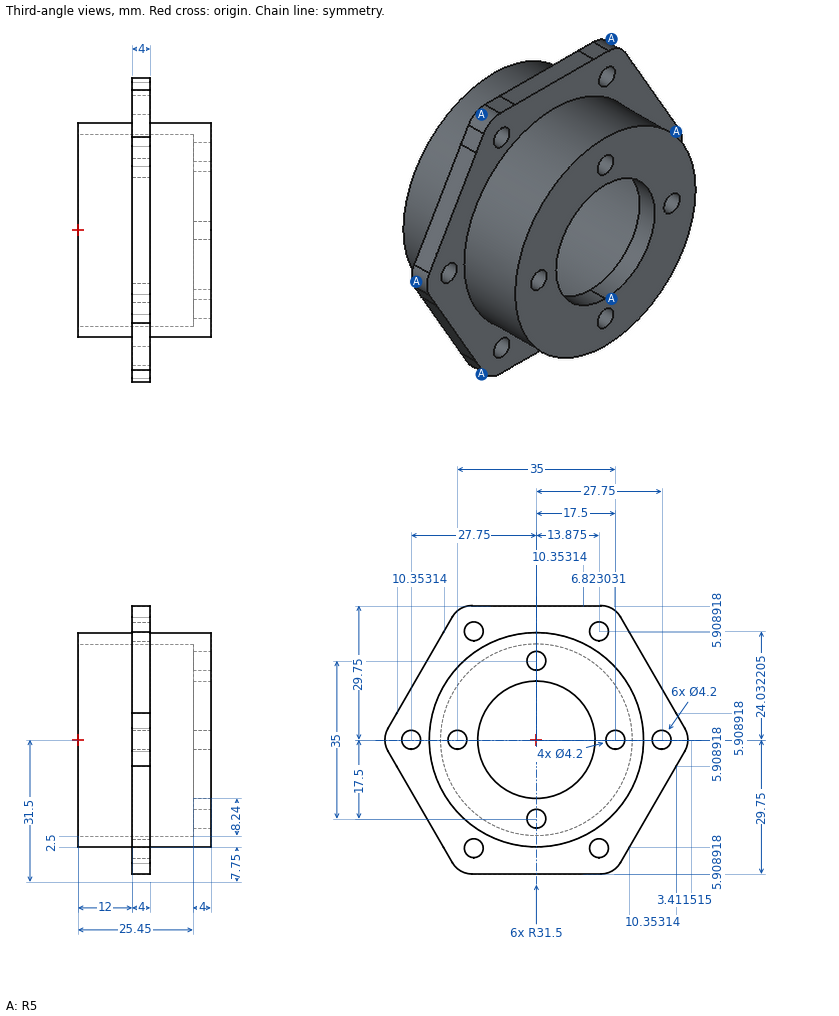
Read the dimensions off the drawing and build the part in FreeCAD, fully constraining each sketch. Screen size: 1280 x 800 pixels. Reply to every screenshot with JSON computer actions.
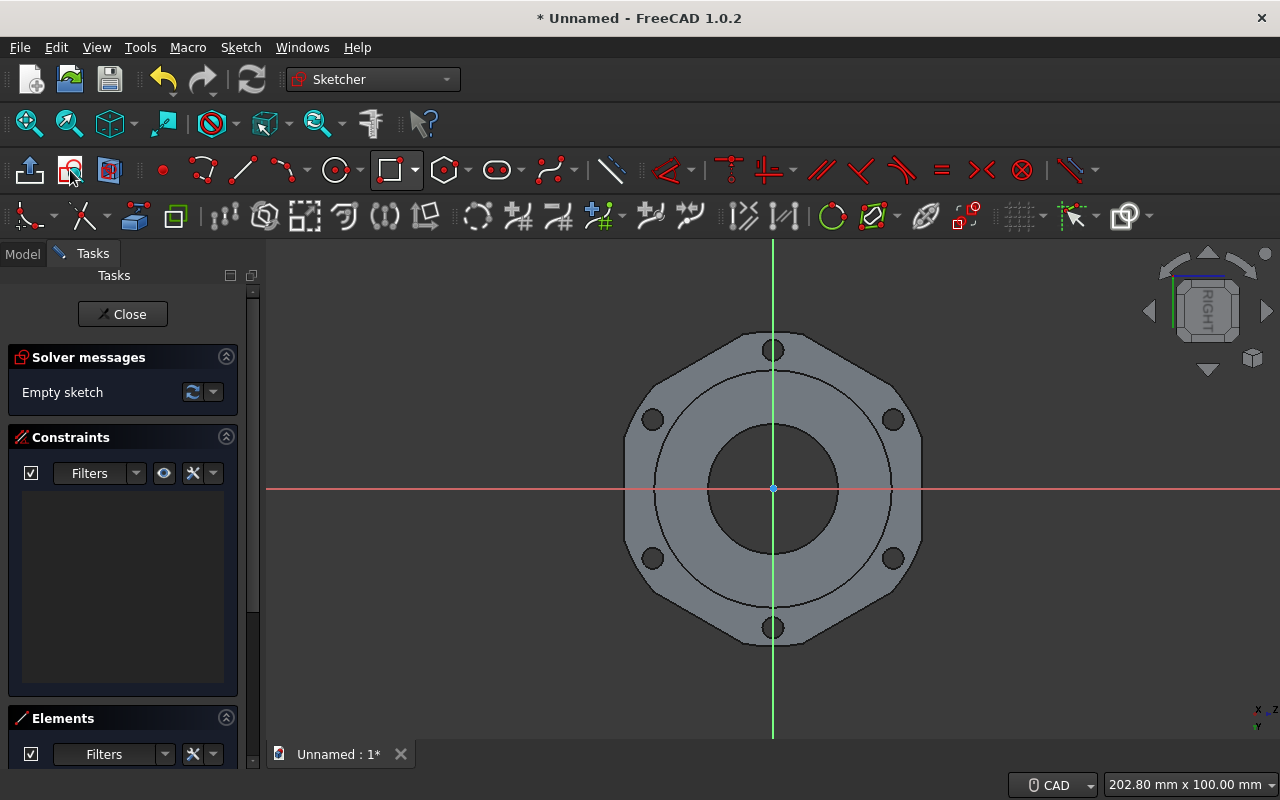
{"action": "scroll", "coordinate": [912, 489], "scroll_direction": "up", "scroll_amount": 2}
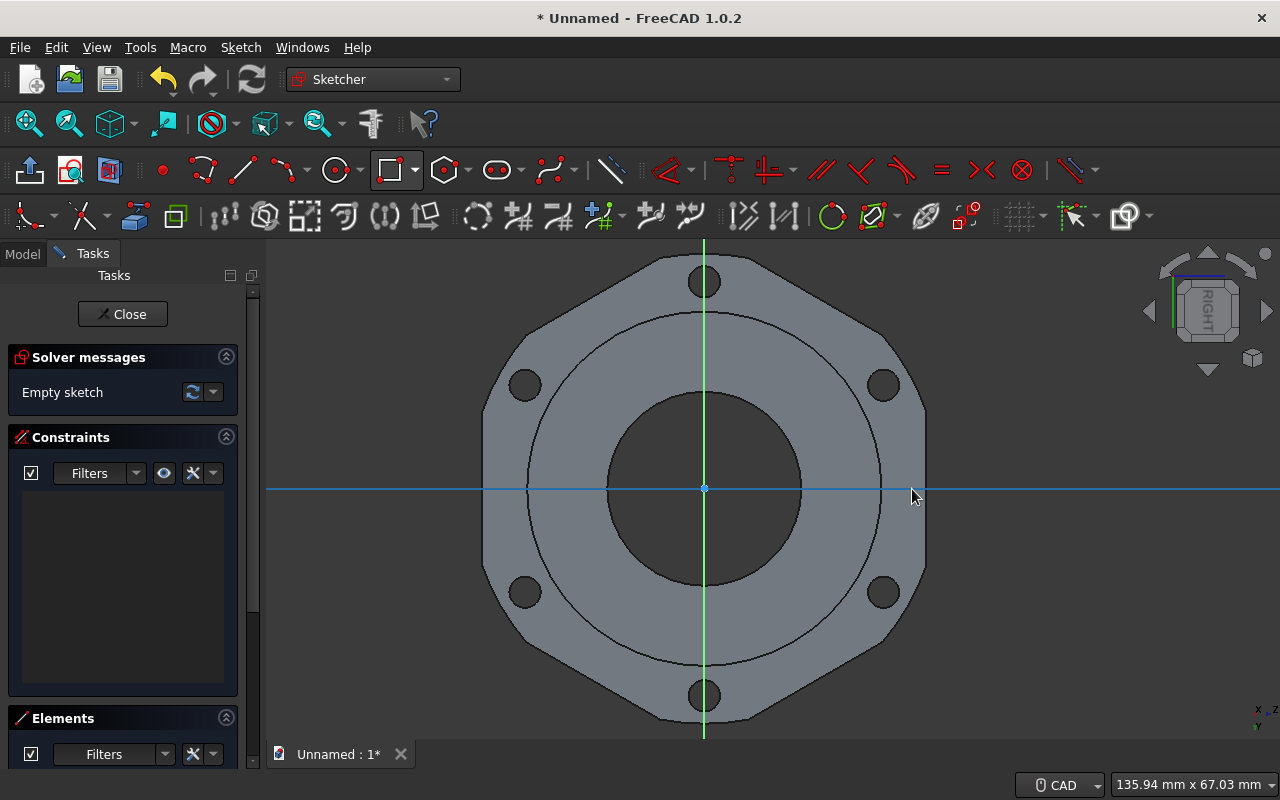
{"action": "key", "text": "g c"}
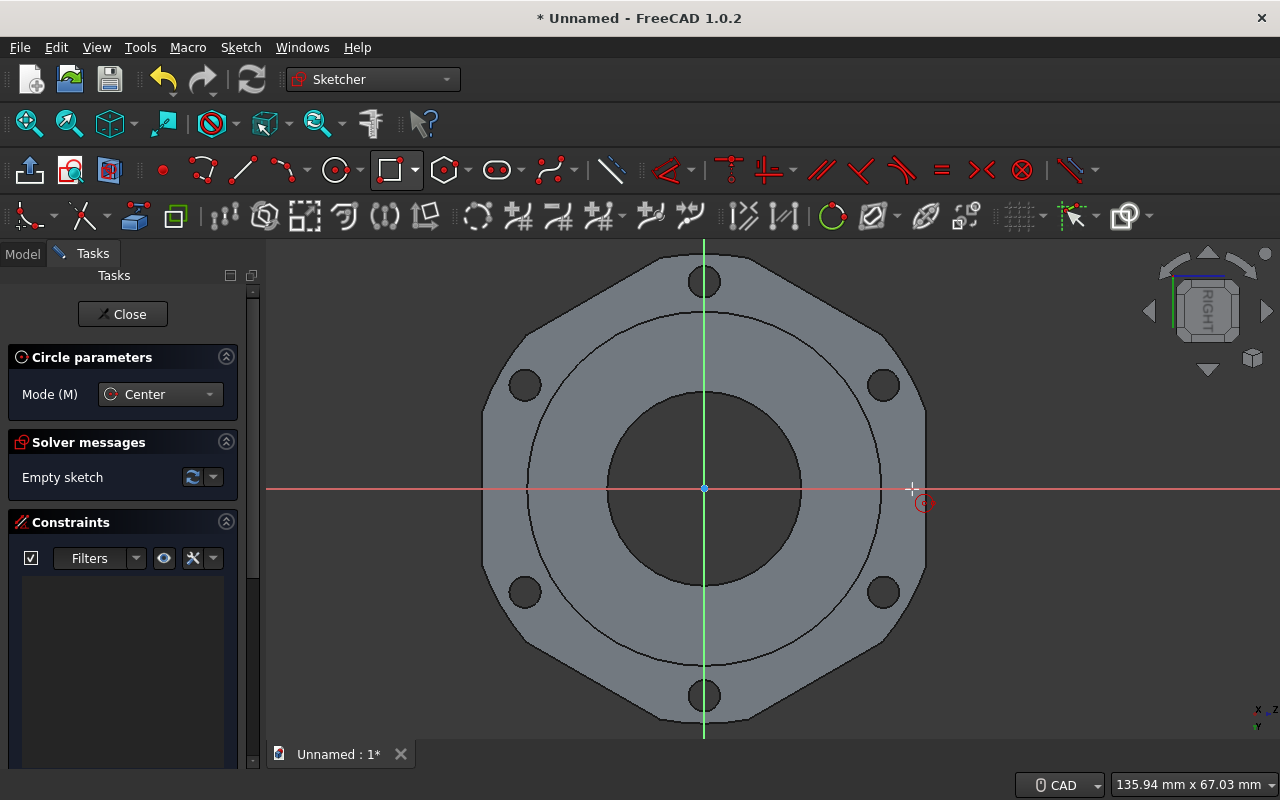
{"action": "scroll", "coordinate": [704, 619], "scroll_direction": "up", "scroll_amount": 2}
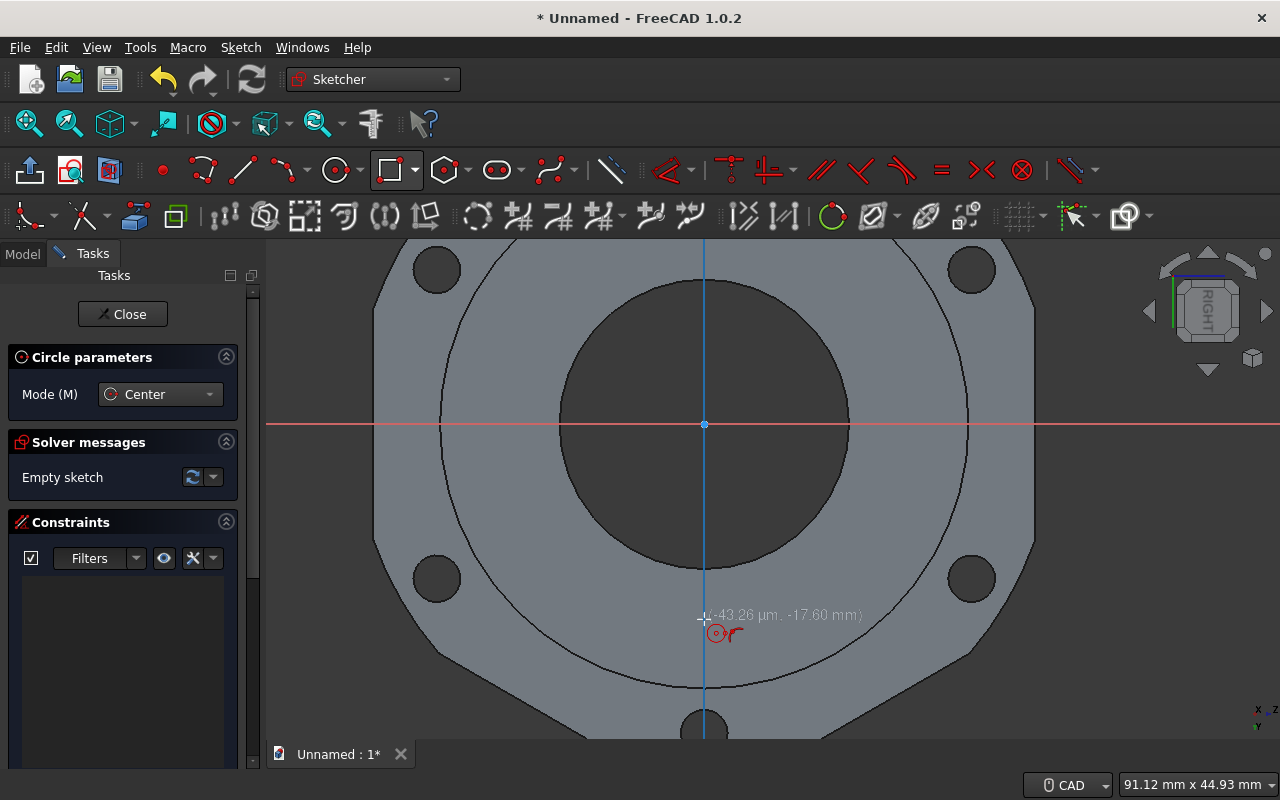
{"action": "left_click", "coordinate": [704, 619]}
{"action": "left_click", "coordinate": [721, 603]}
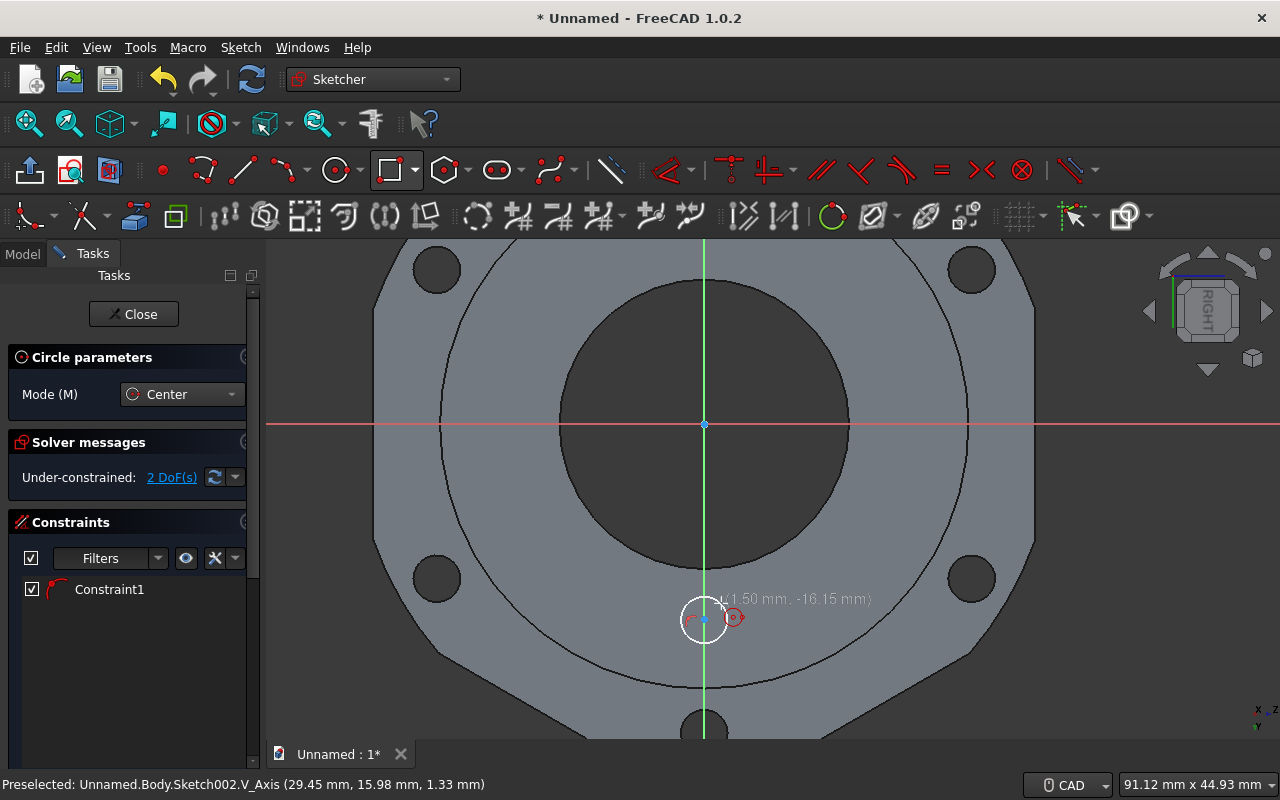
{"action": "left_click", "coordinate": [510, 424]}
{"action": "left_click", "coordinate": [526, 408]}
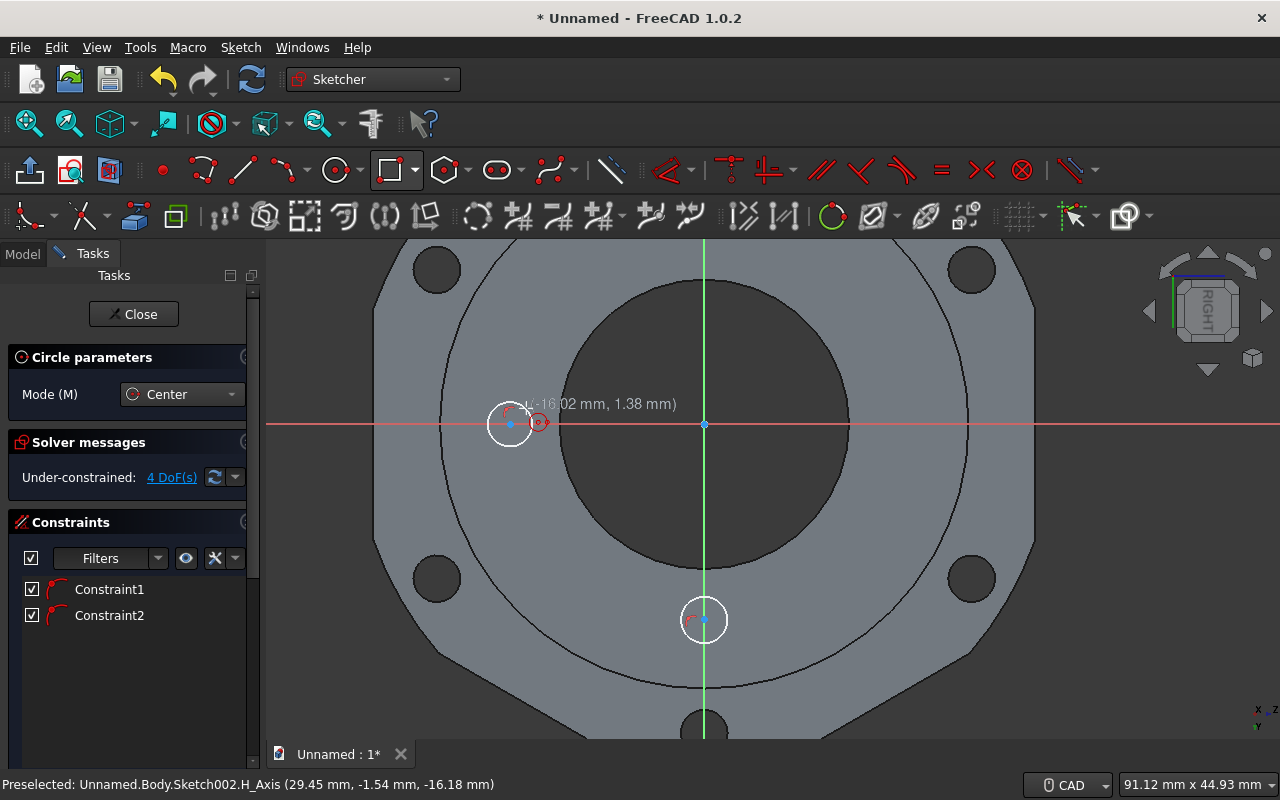
{"action": "scroll", "coordinate": [705, 621], "scroll_direction": "down", "scroll_amount": 2}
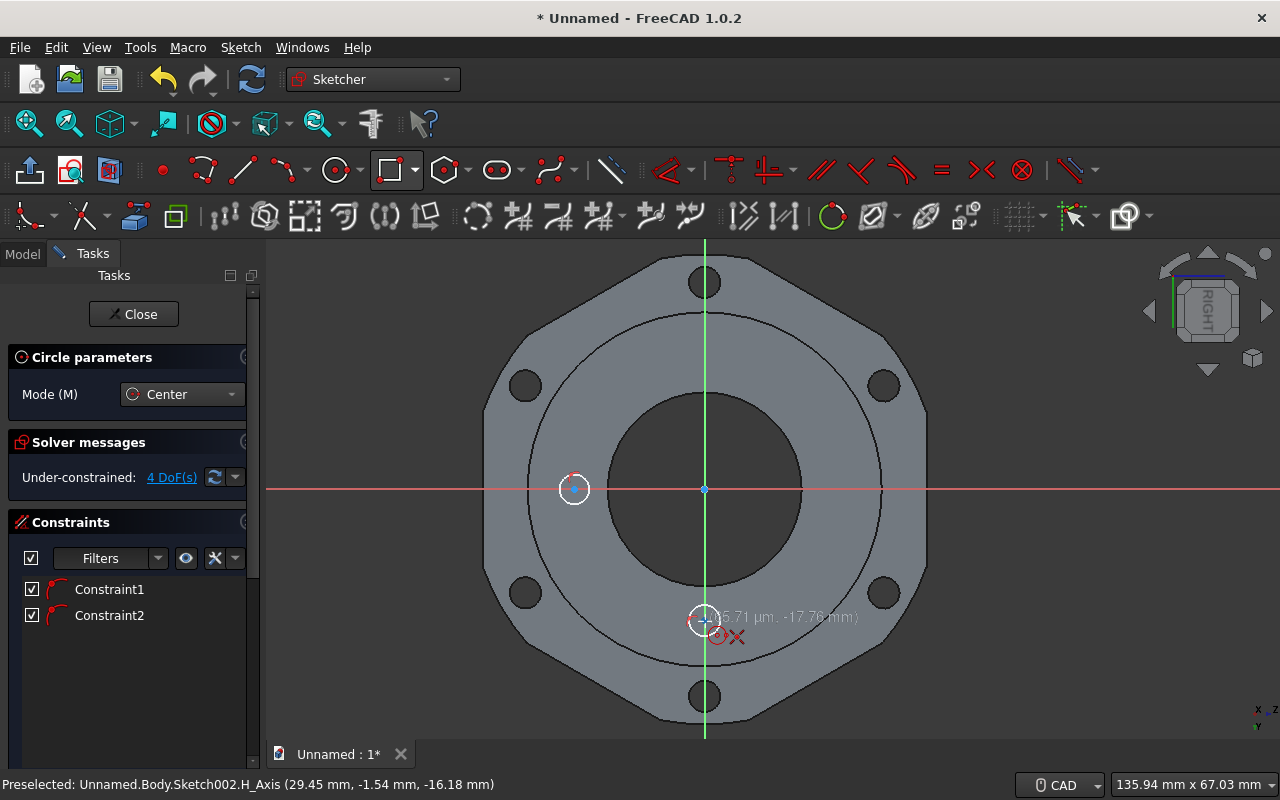
{"action": "scroll", "coordinate": [705, 359], "scroll_direction": "up", "scroll_amount": 2}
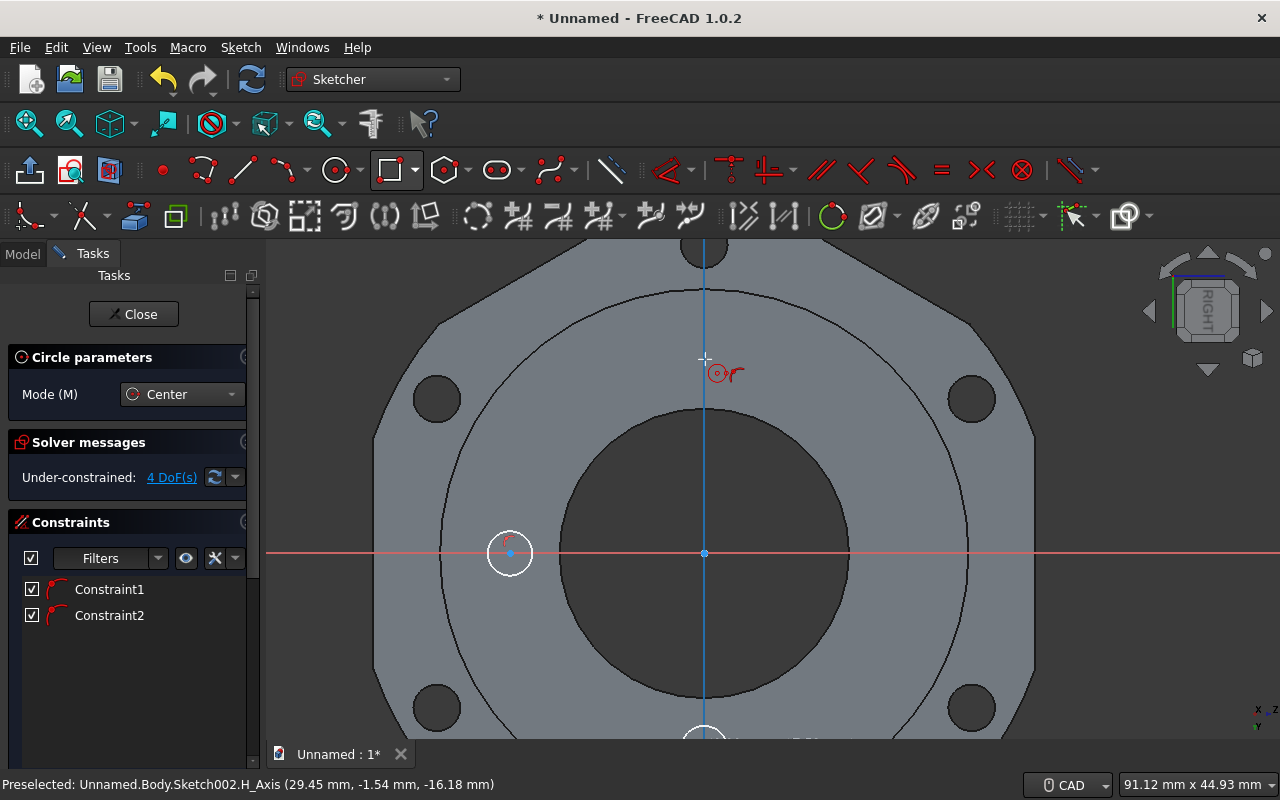
{"action": "left_click", "coordinate": [704, 359]}
{"action": "left_click", "coordinate": [721, 342]}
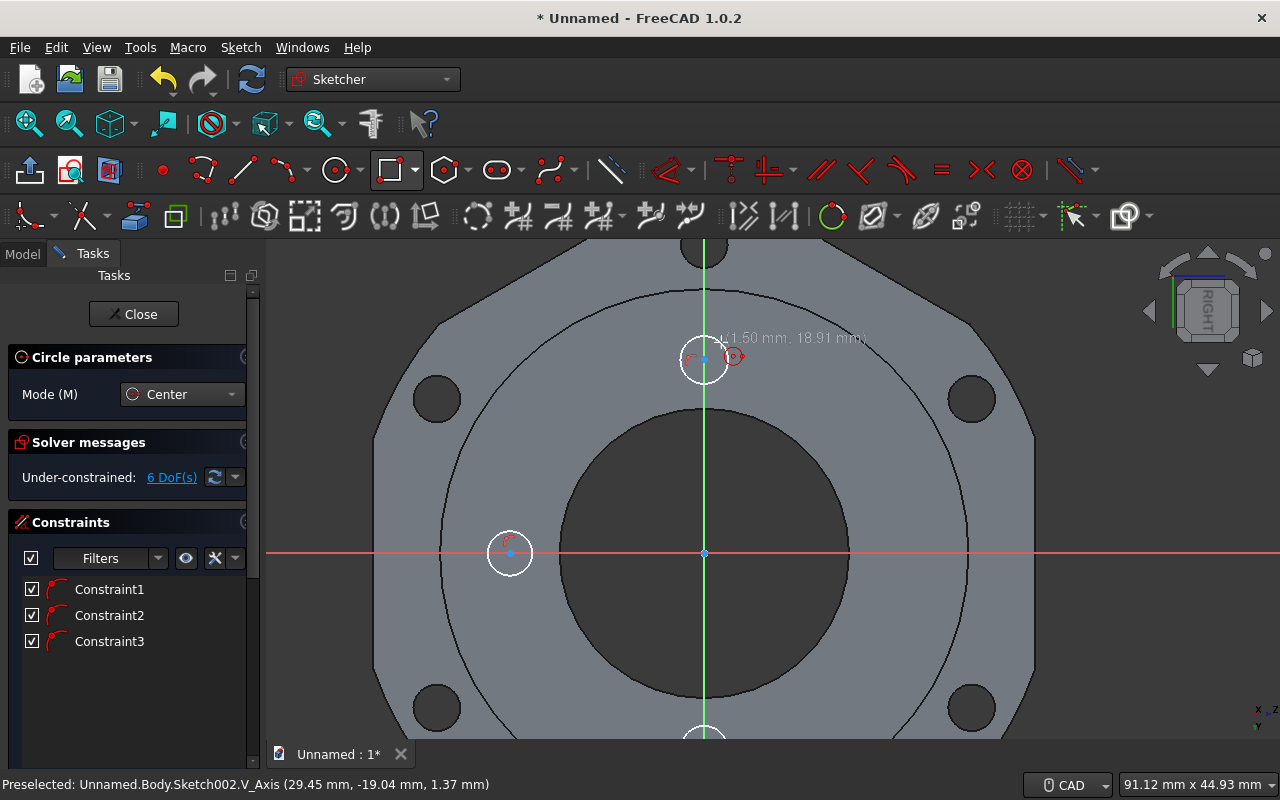
{"action": "left_click", "coordinate": [899, 553]}
{"action": "left_click", "coordinate": [916, 537]}
{"action": "key", "text": "Escape"}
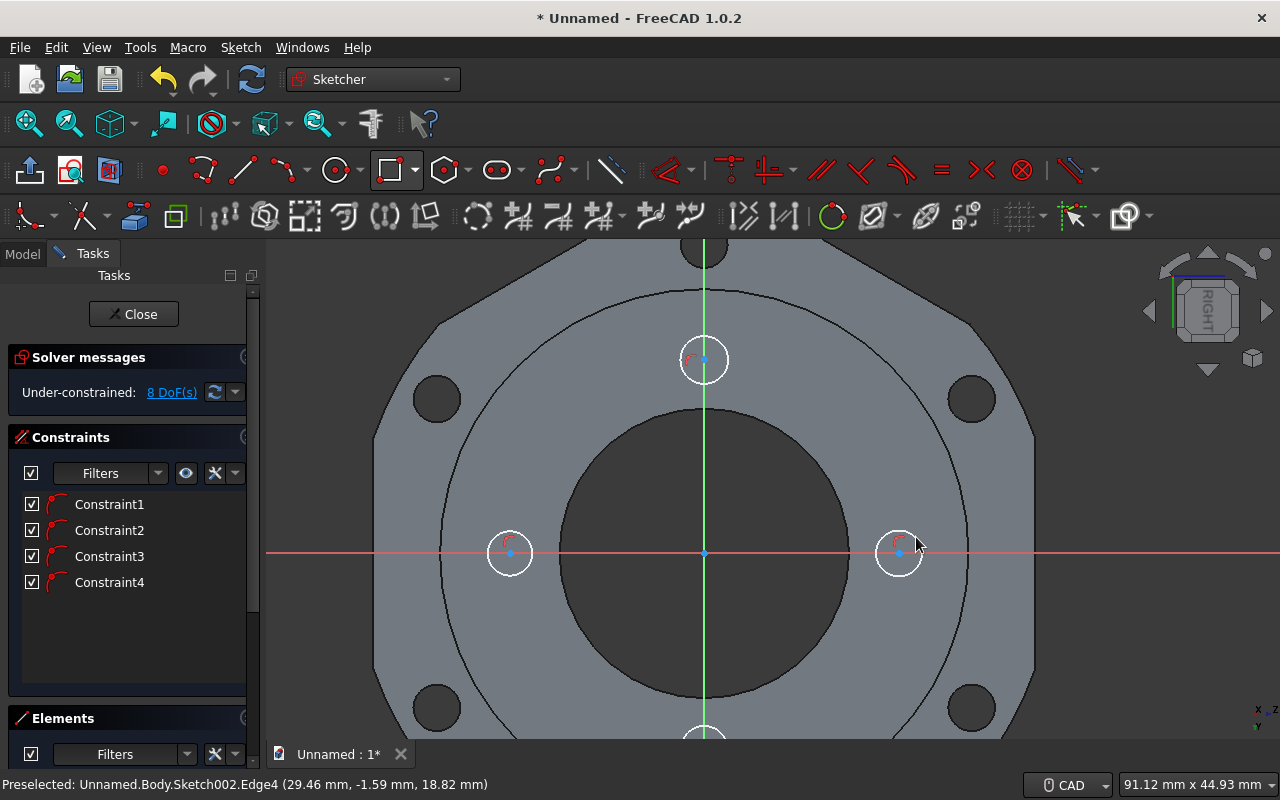
{"action": "scroll", "coordinate": [705, 358], "scroll_direction": "down", "scroll_amount": 2}